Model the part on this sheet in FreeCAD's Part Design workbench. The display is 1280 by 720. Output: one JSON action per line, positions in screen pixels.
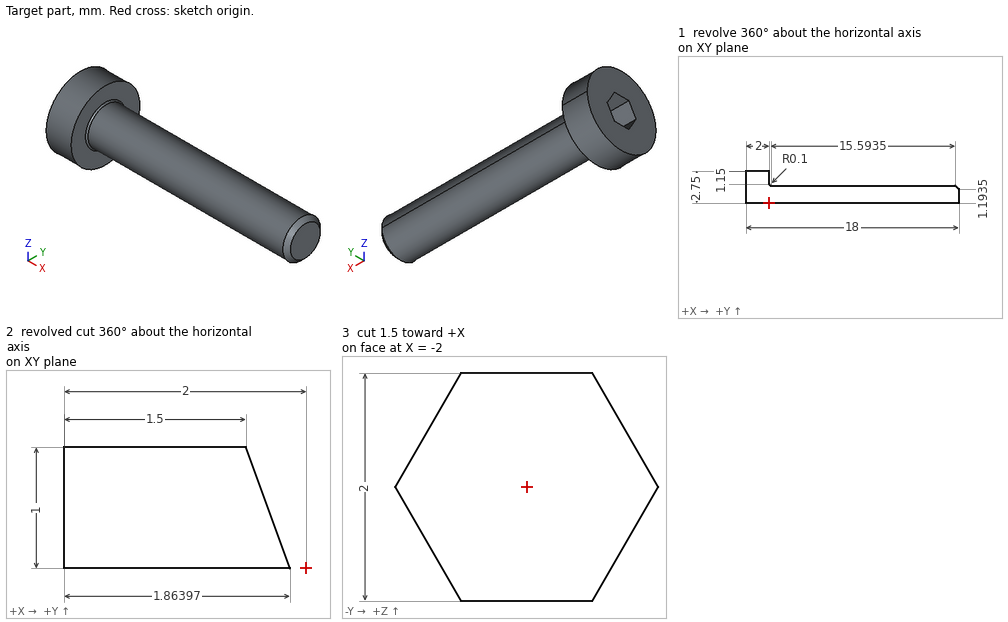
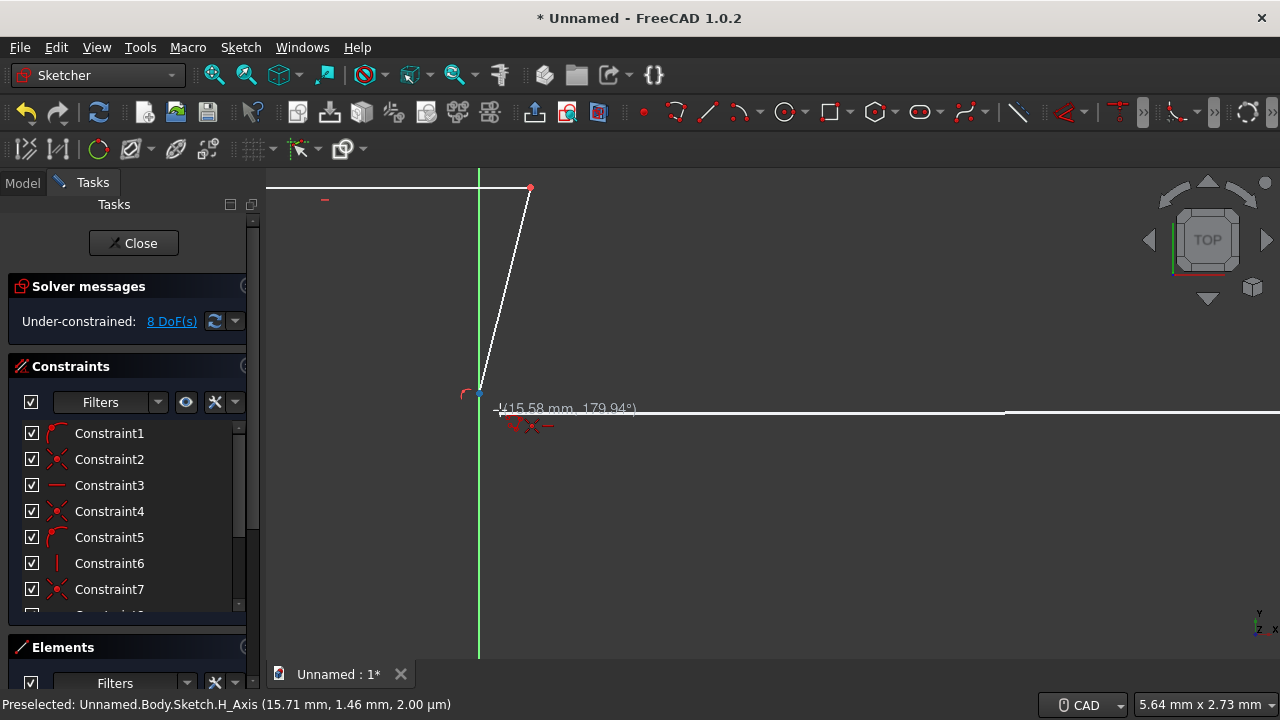
{"action": "left_click", "coordinate": [497, 406]}
{"action": "right_click", "coordinate": [497, 406]}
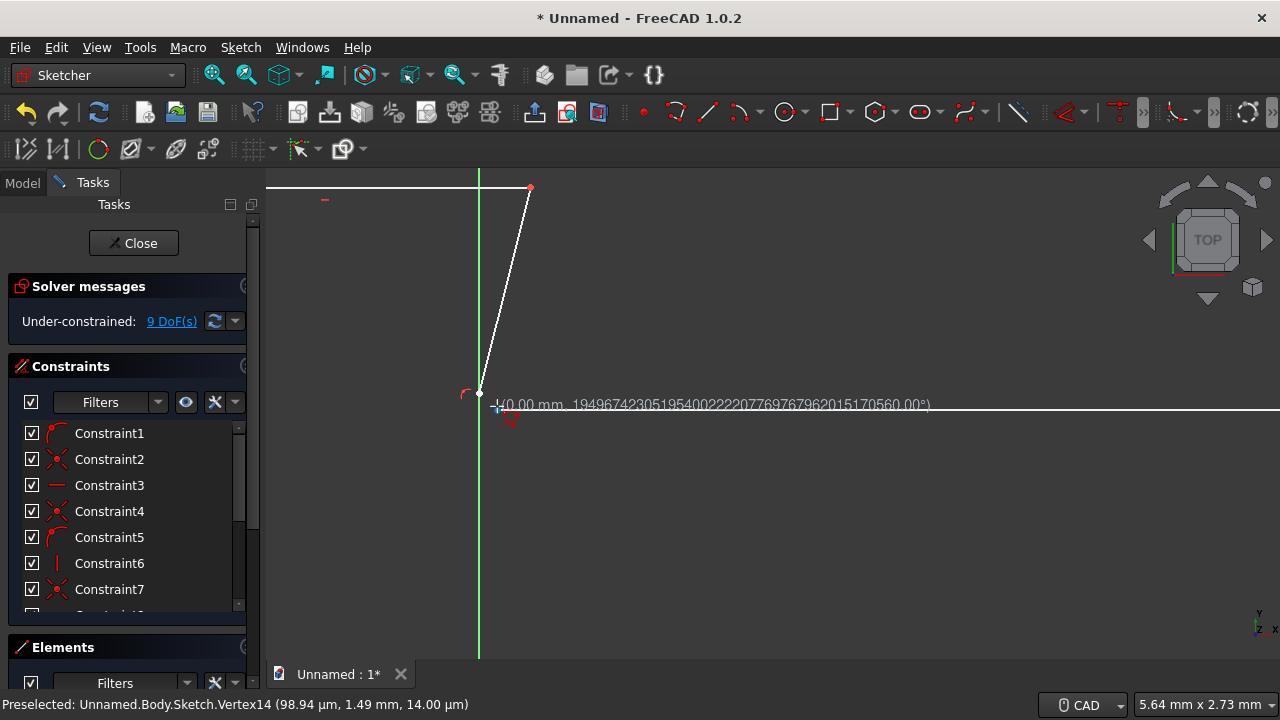
{"action": "key", "text": "g 3 a"}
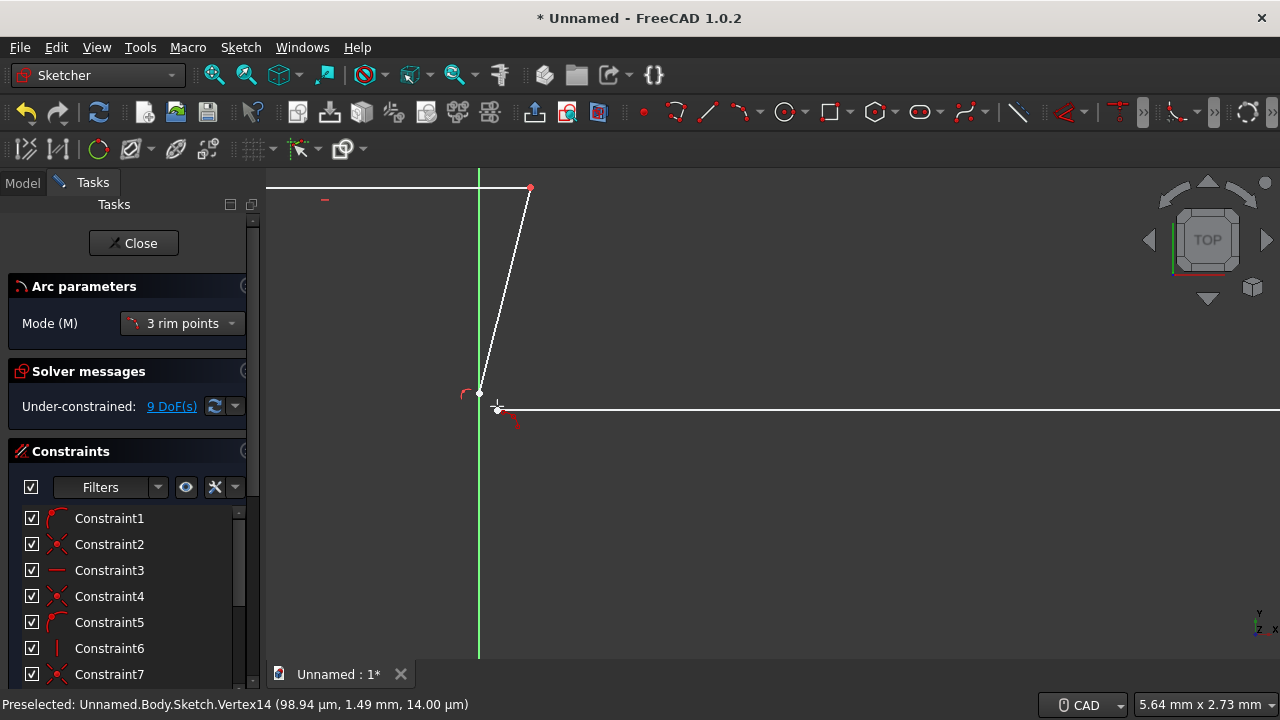
{"action": "left_click", "coordinate": [497, 410]}
{"action": "left_click", "coordinate": [479, 393]}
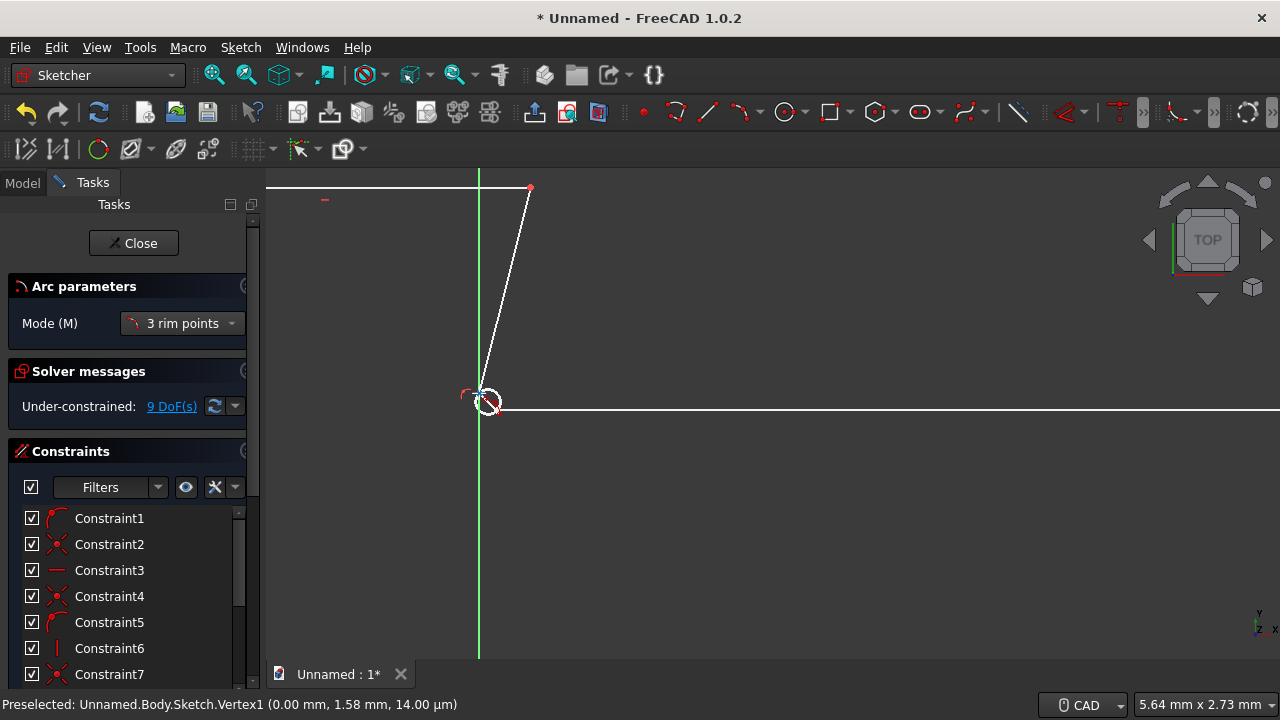
{"action": "scroll", "coordinate": [484, 403], "scroll_direction": "up", "scroll_amount": 6}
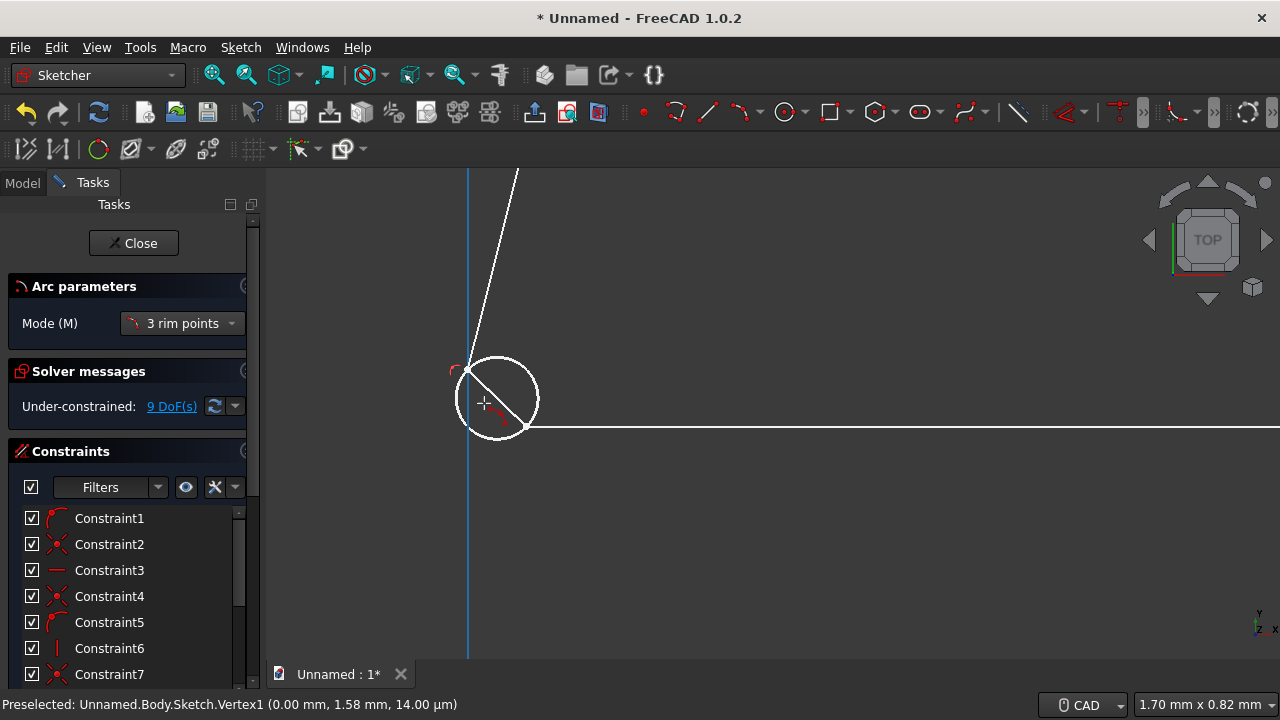
{"action": "left_click", "coordinate": [485, 401]}
{"action": "key", "text": "Escape"}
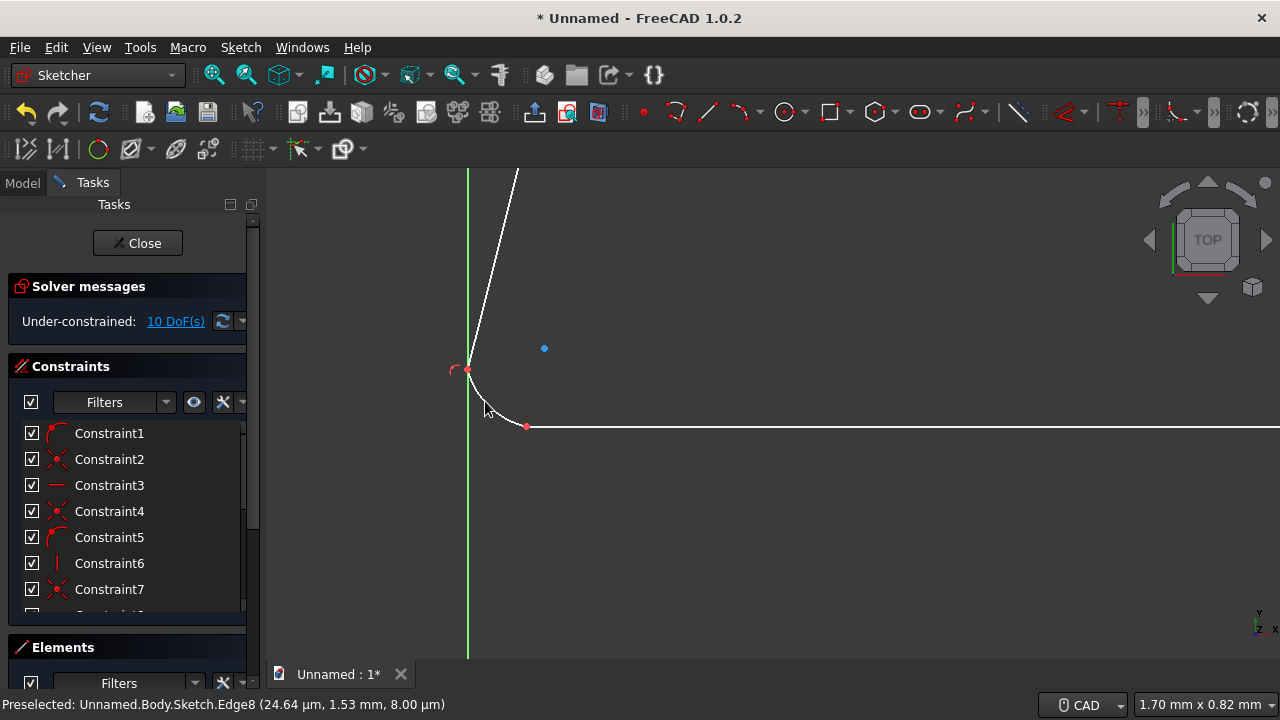
{"action": "left_click", "coordinate": [502, 233]}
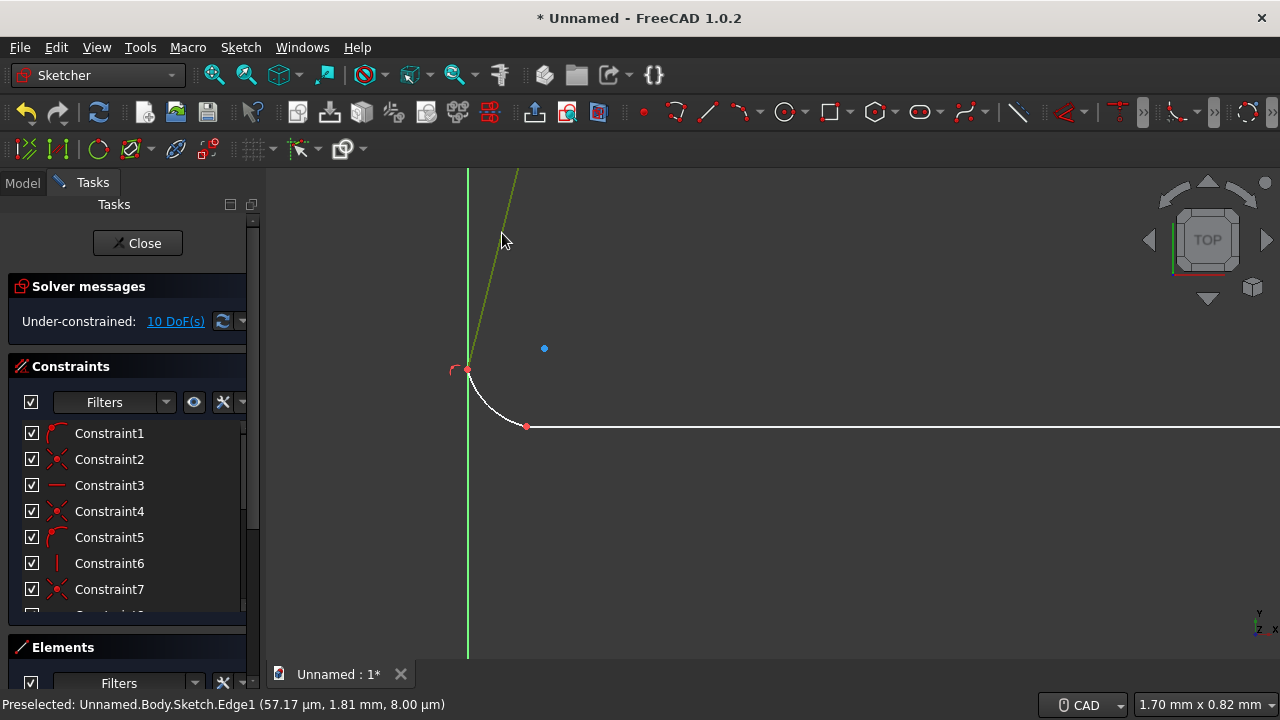
{"action": "left_click", "coordinate": [478, 393]}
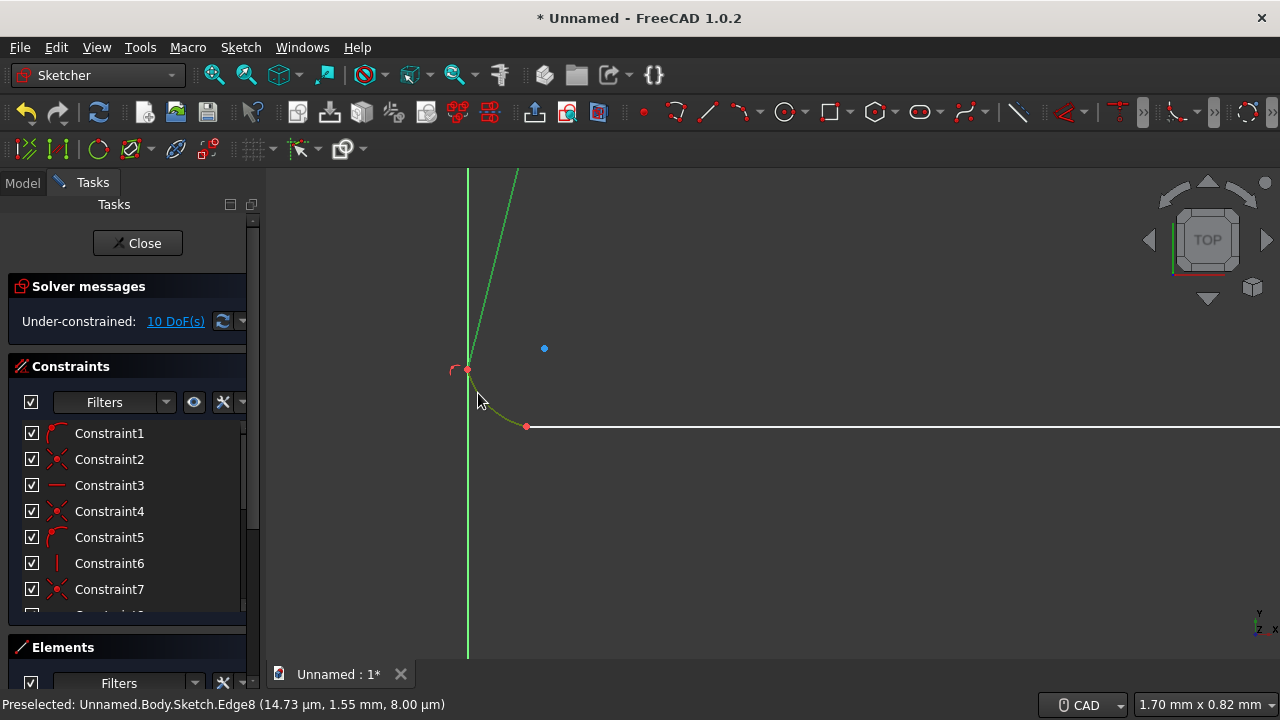
{"action": "key", "text": "t"}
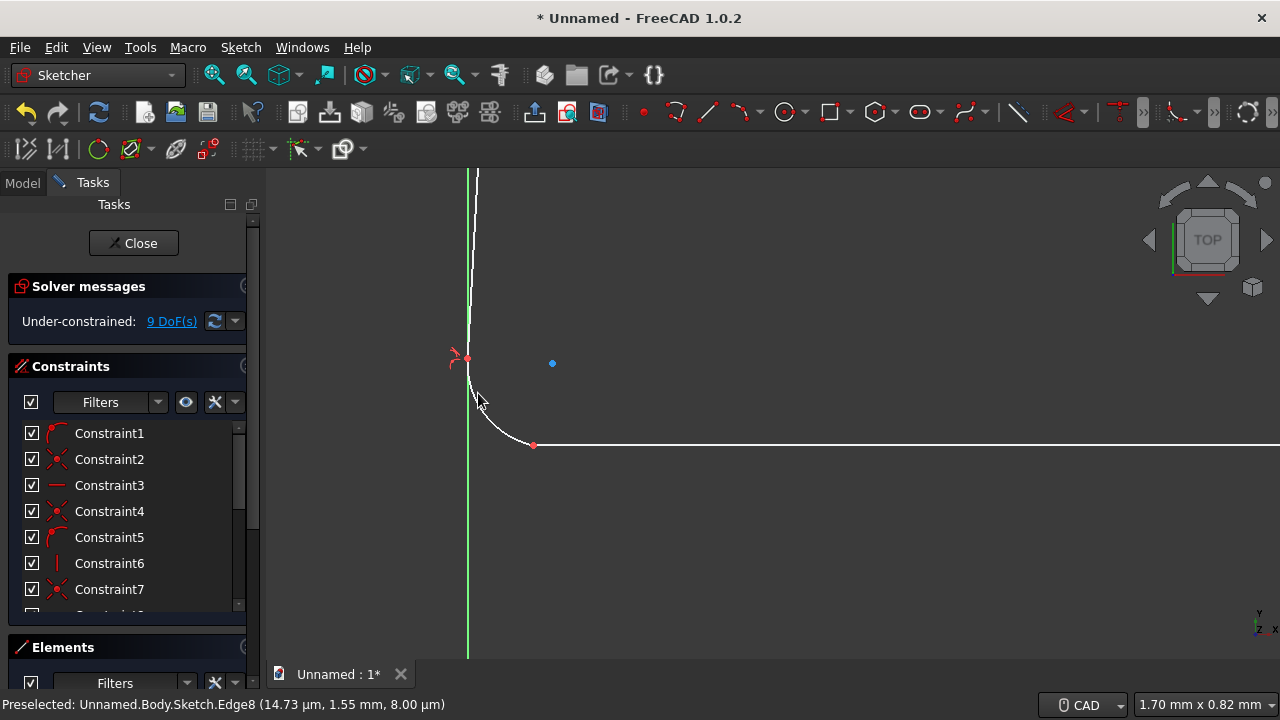
{"action": "scroll", "coordinate": [498, 409], "scroll_direction": "down", "scroll_amount": 15}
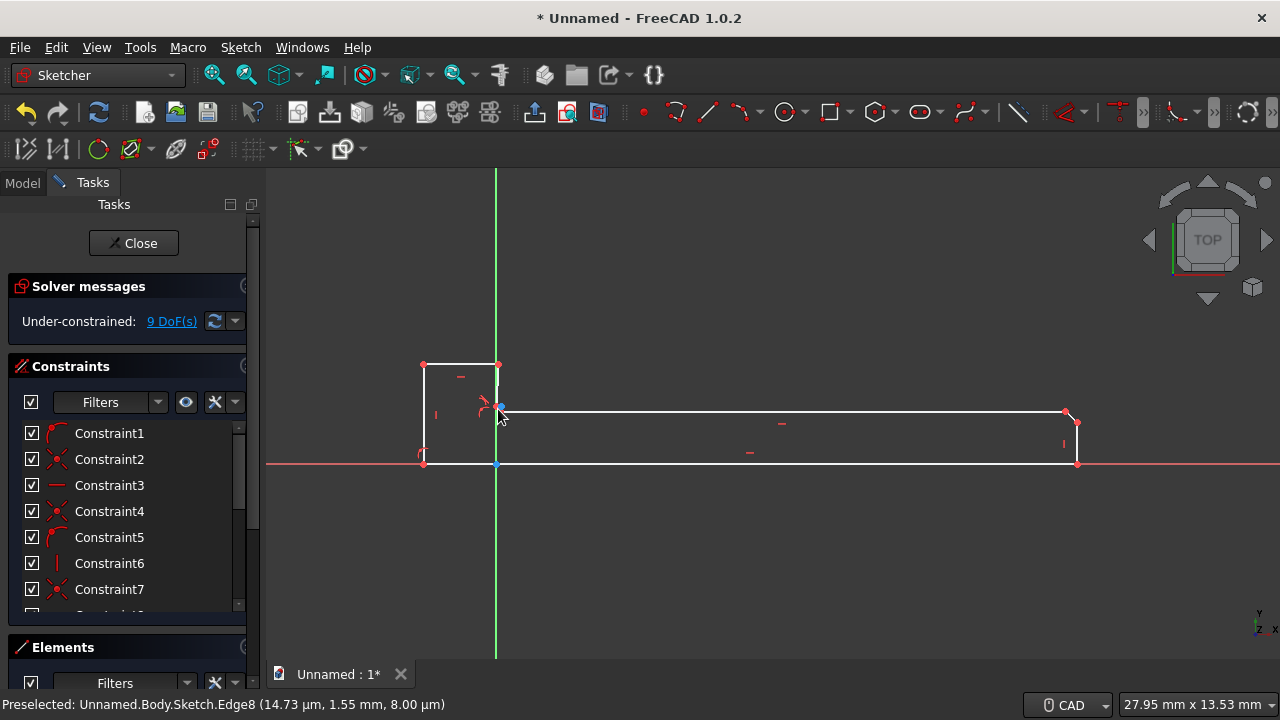
{"action": "left_click", "coordinate": [824, 411]}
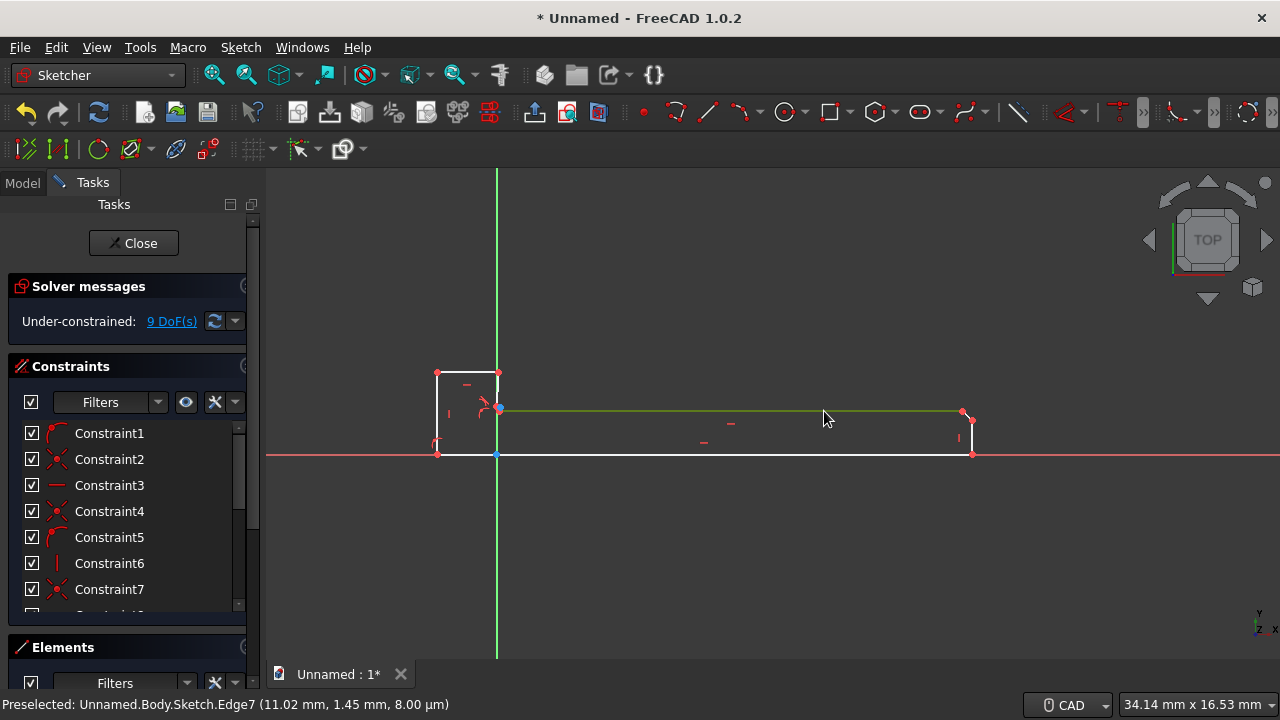
{"action": "scroll", "coordinate": [498, 410], "scroll_direction": "up", "scroll_amount": 8}